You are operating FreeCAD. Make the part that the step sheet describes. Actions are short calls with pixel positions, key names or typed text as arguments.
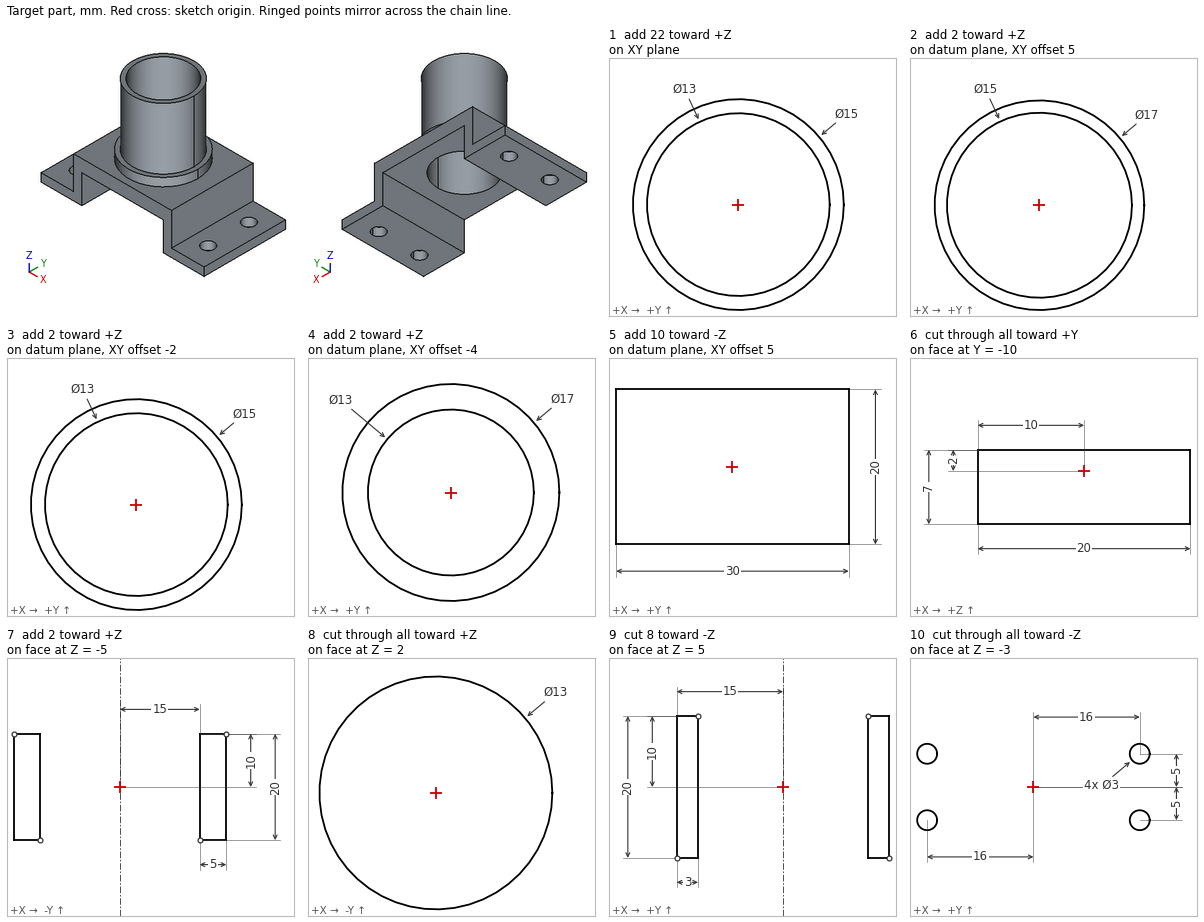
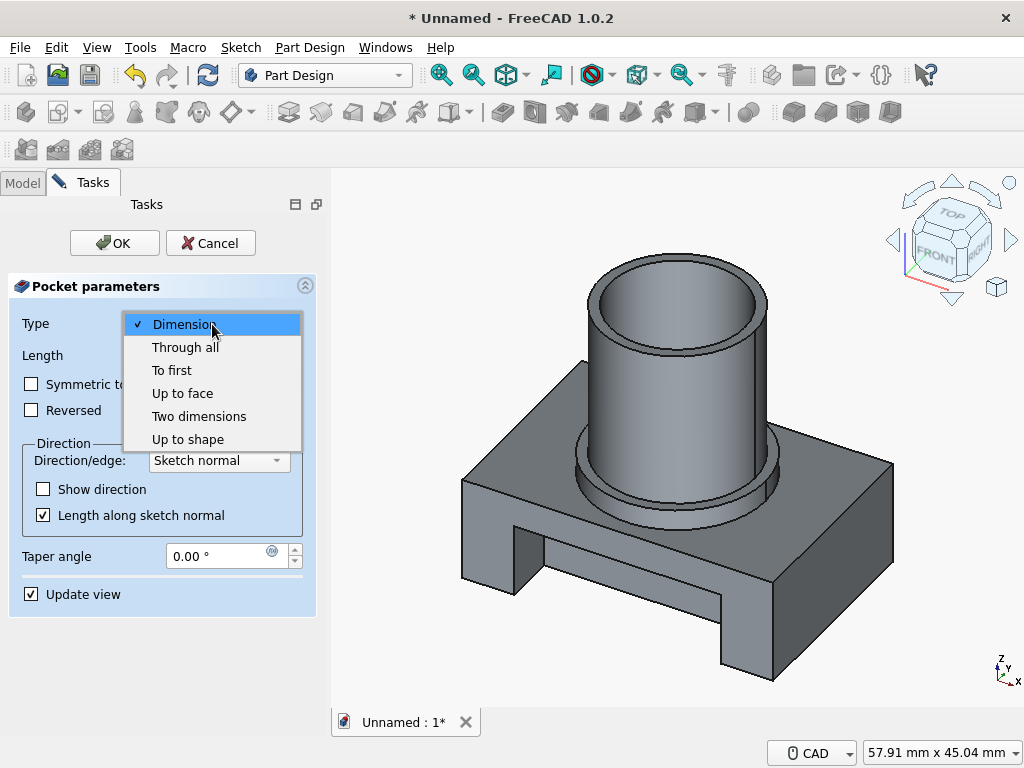
click(212, 348)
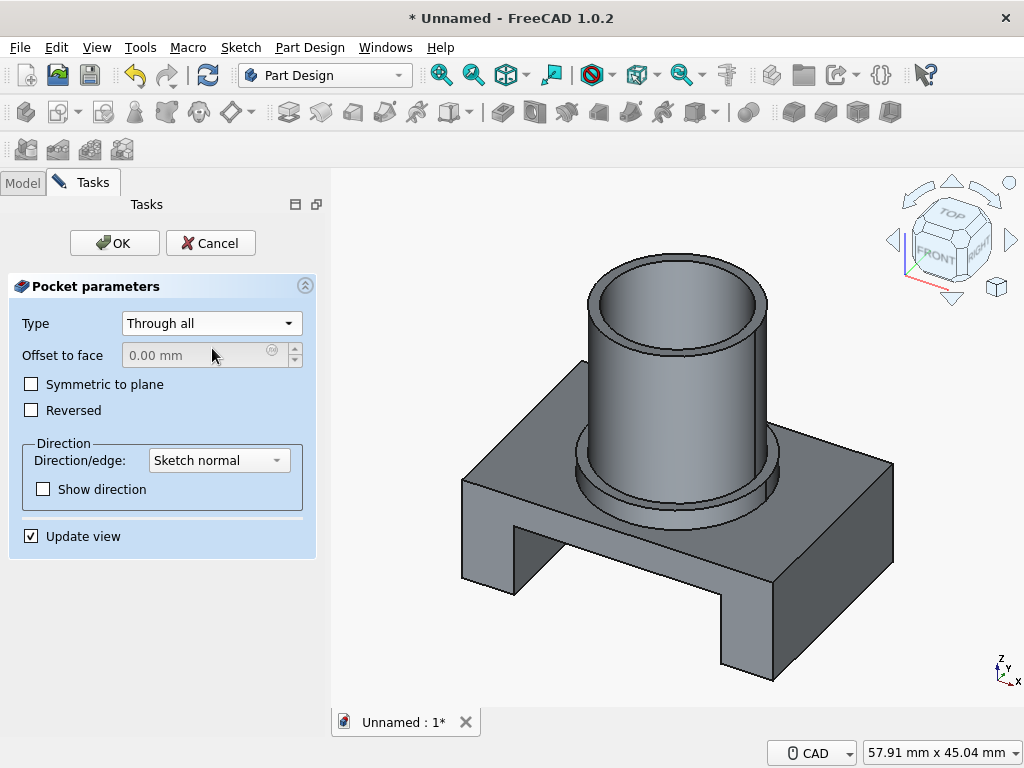
click(115, 243)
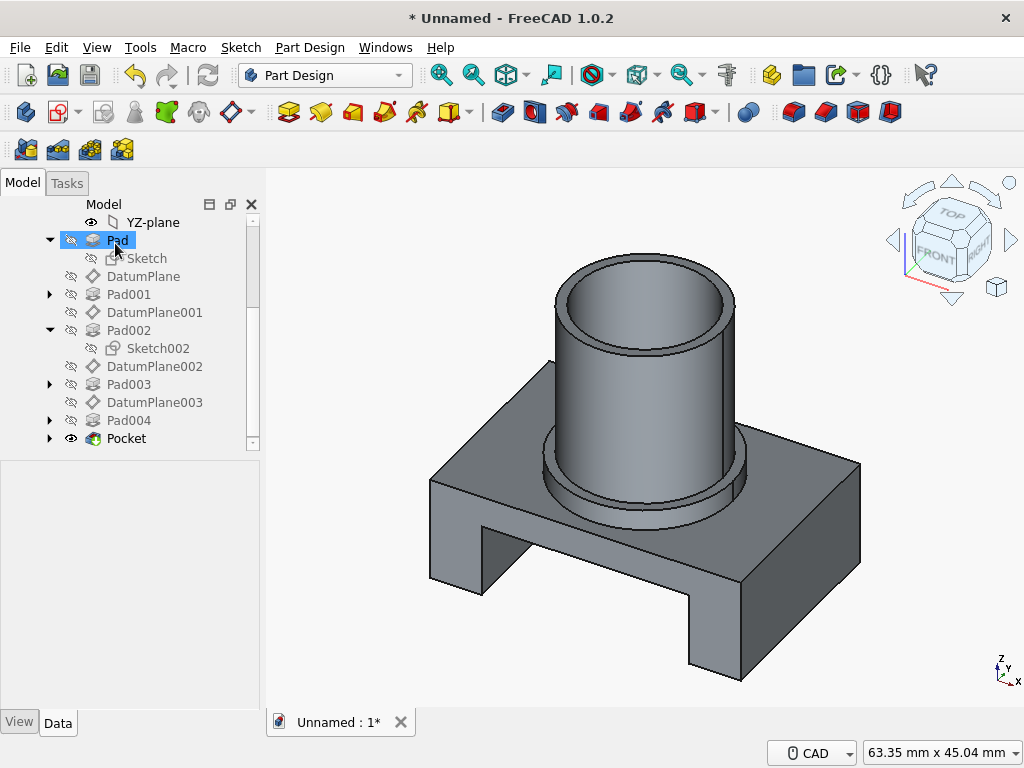
key(5)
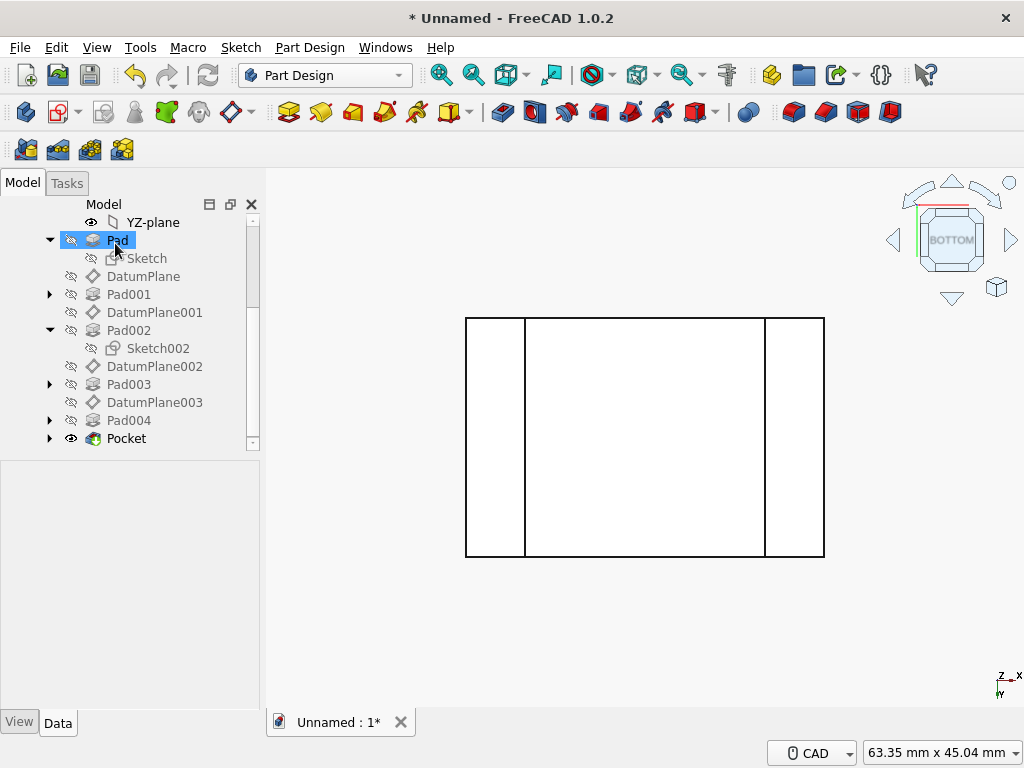
click(795, 505)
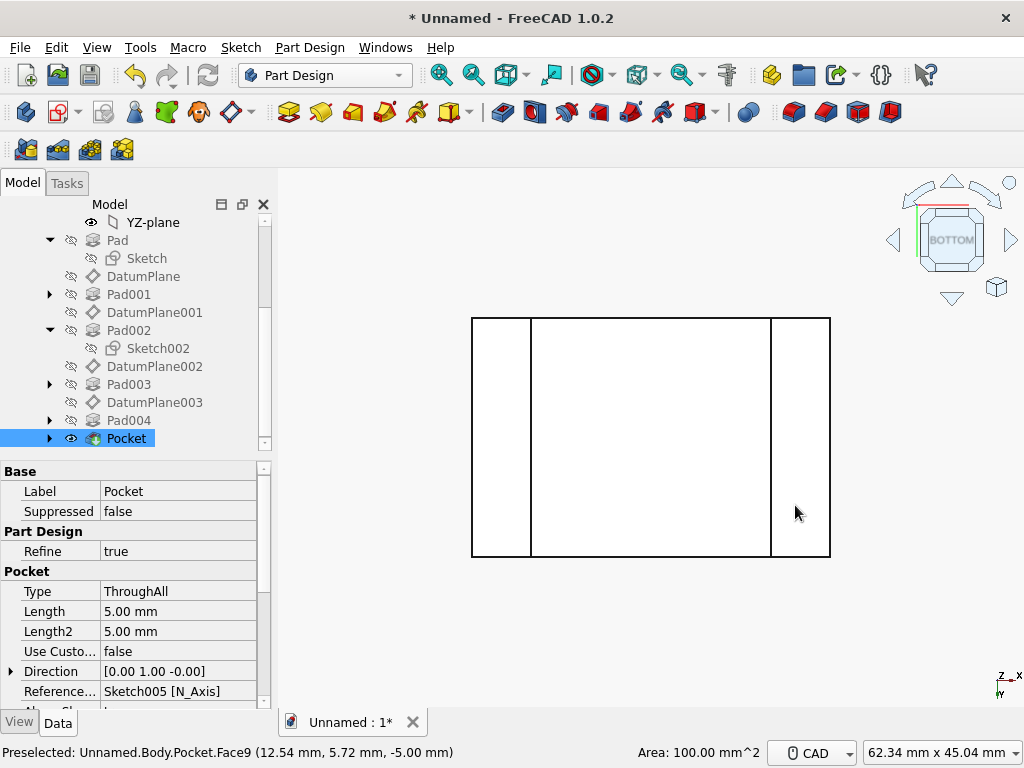
click(58, 112)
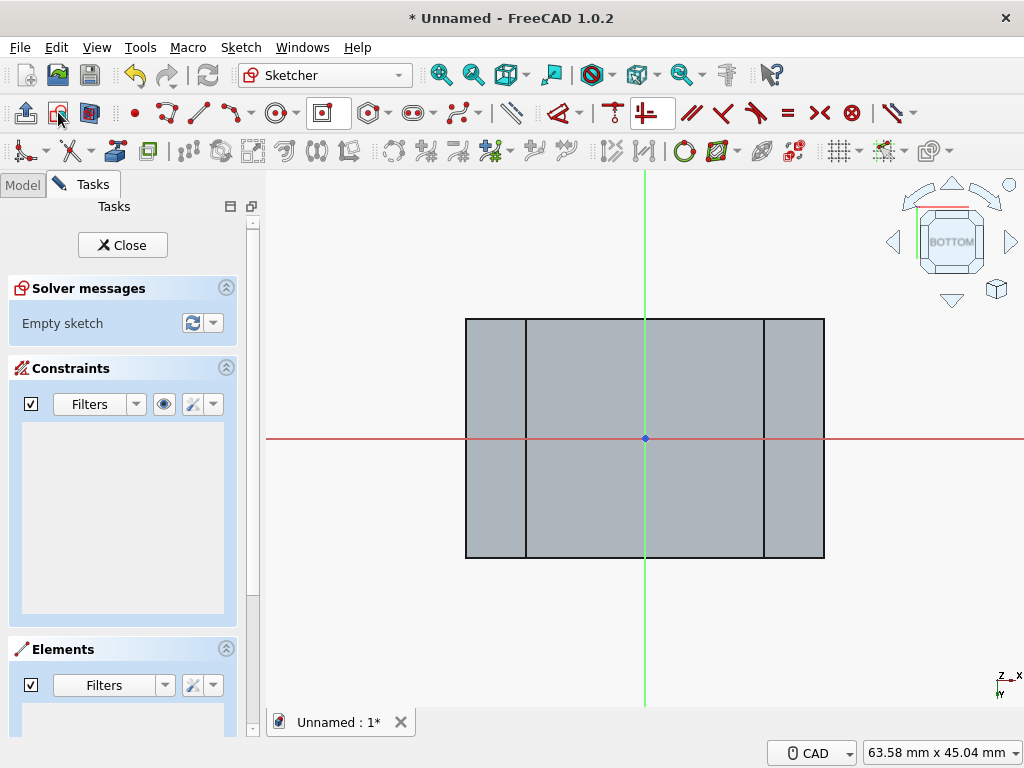
scroll(294, 439, down, 1)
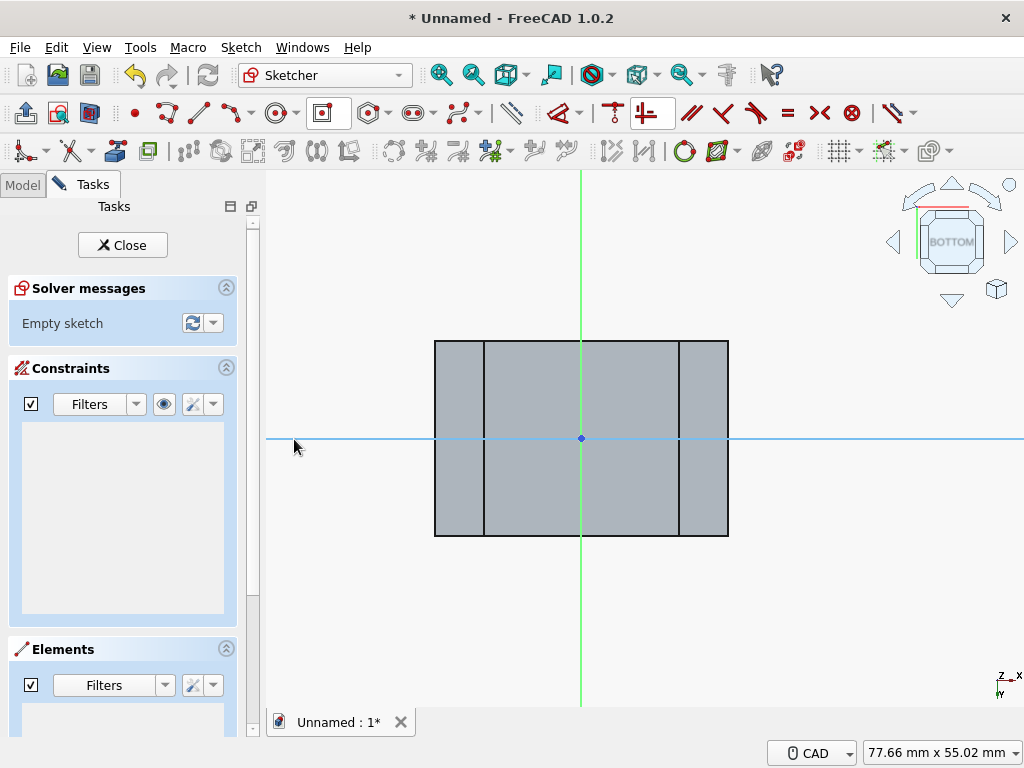
key(g)
key(r)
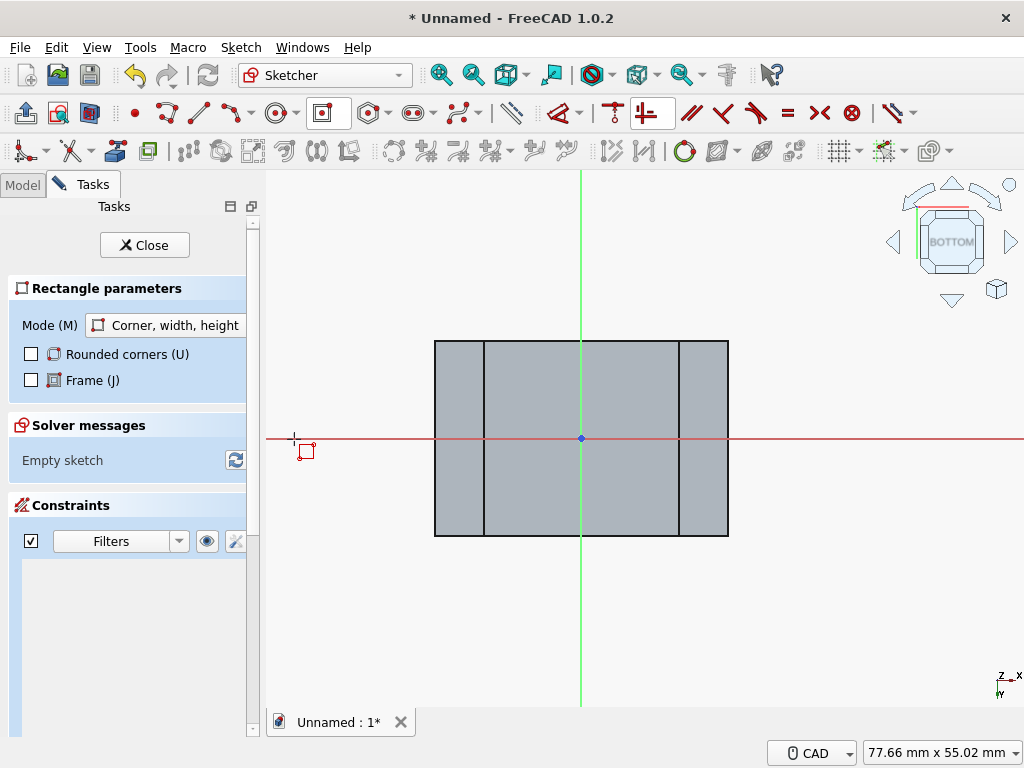
click(728, 341)
click(777, 536)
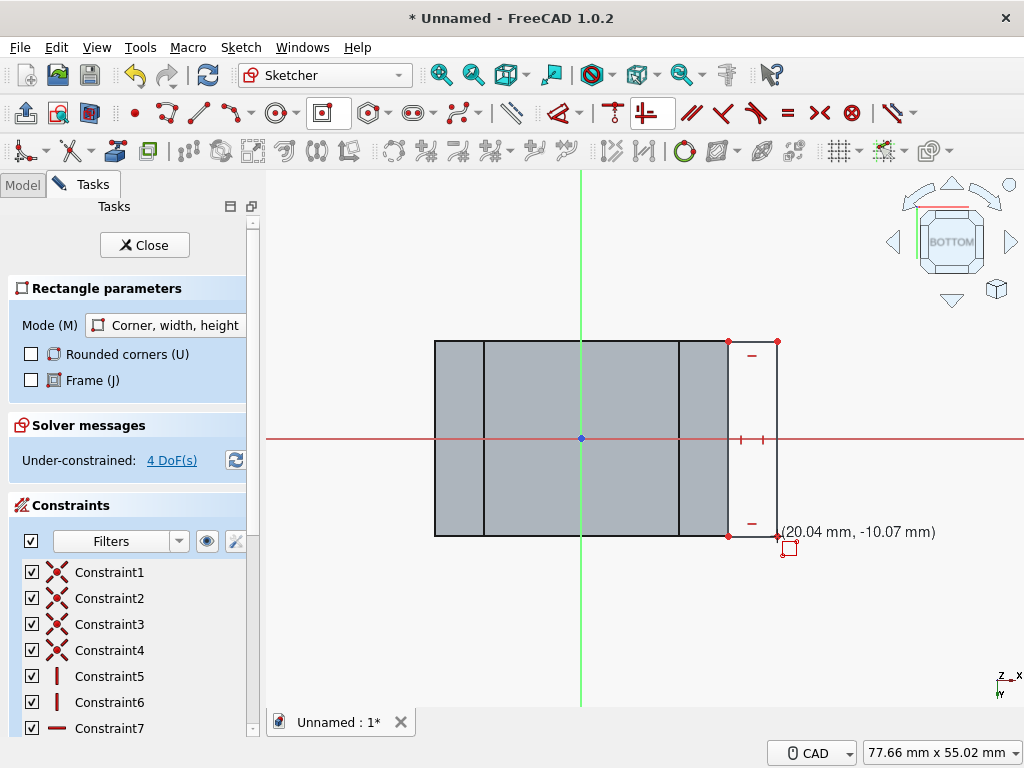
click(386, 341)
click(435, 536)
key(Escape)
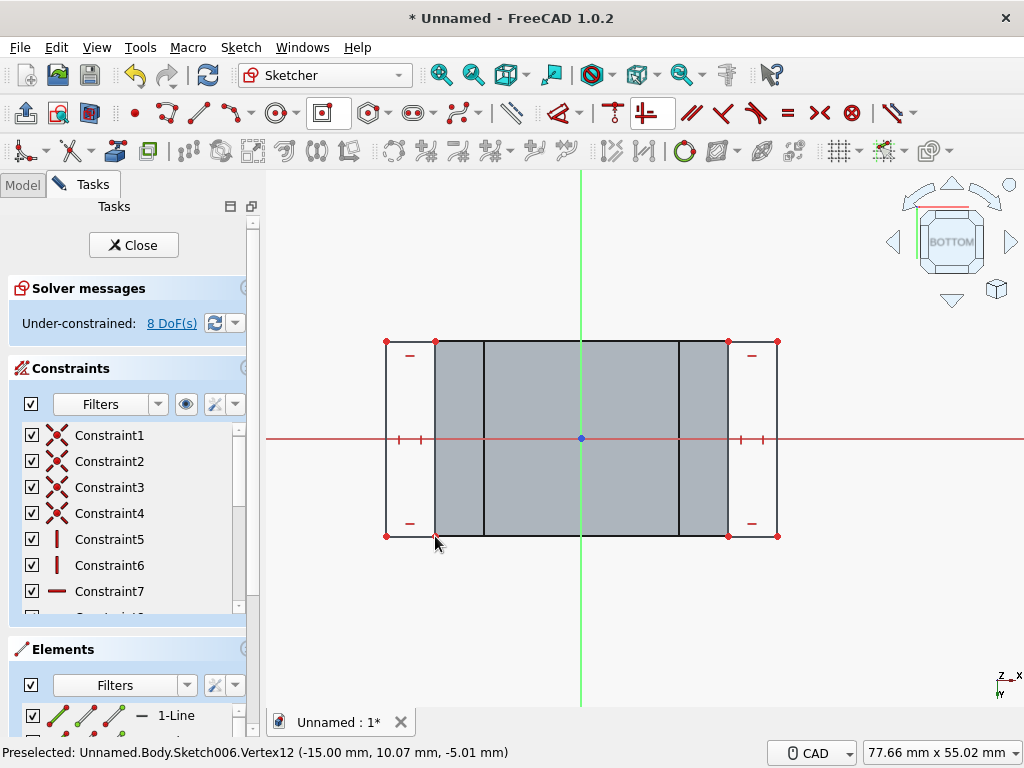
click(777, 342)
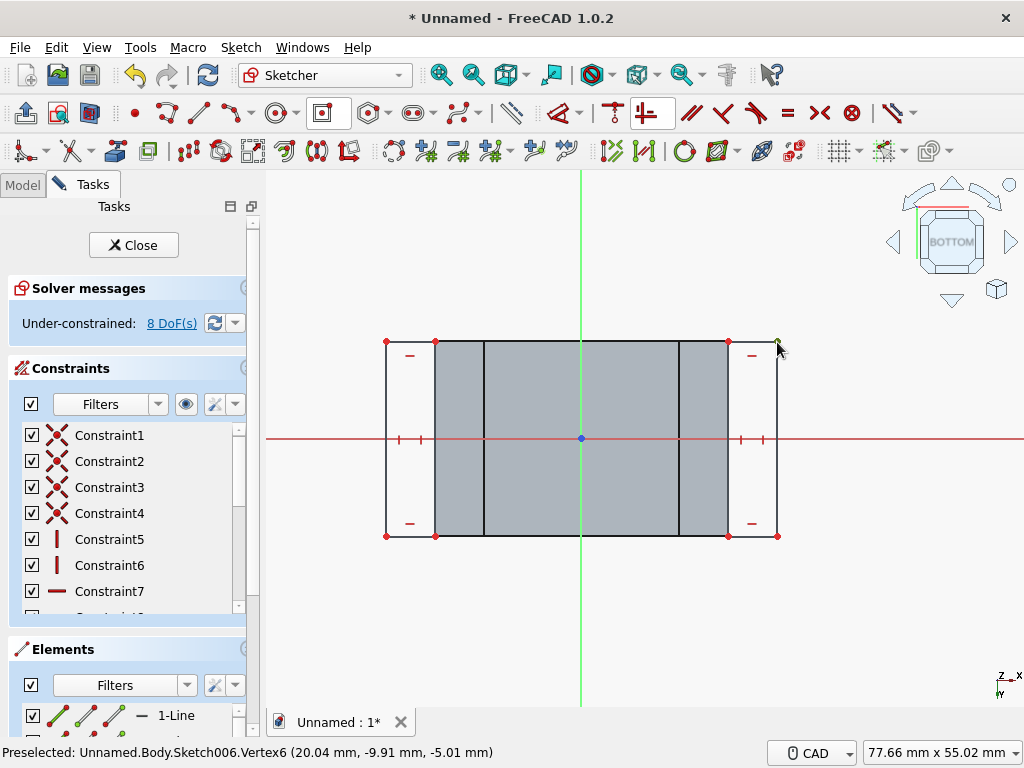
click(386, 342)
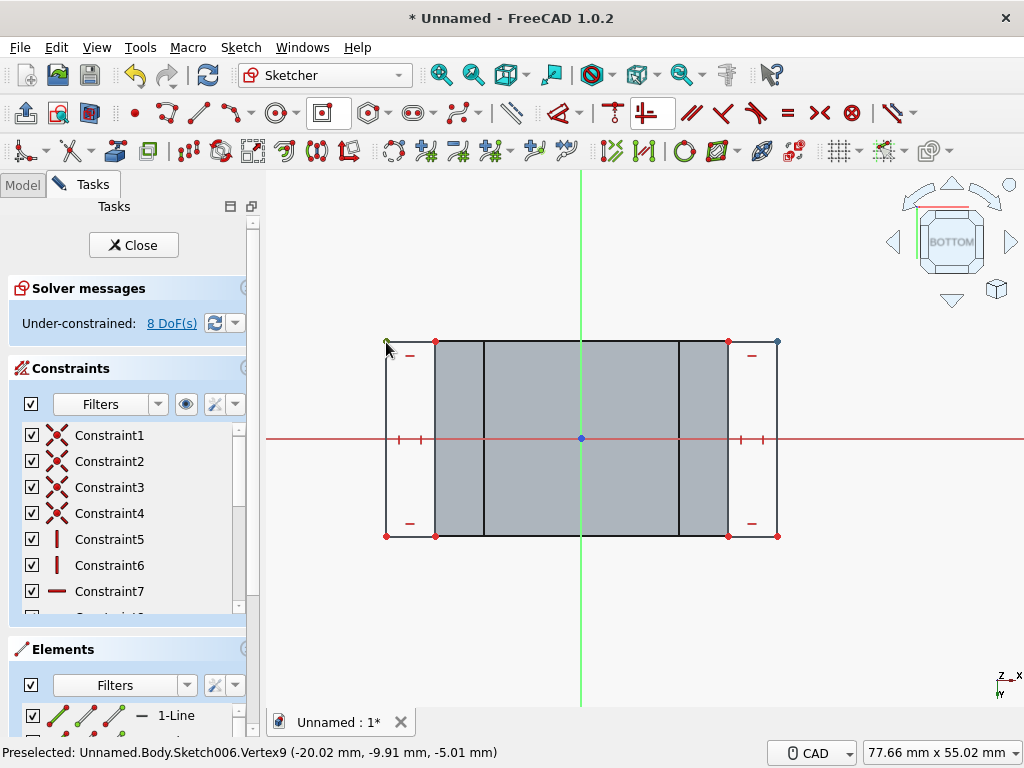
click(581, 645)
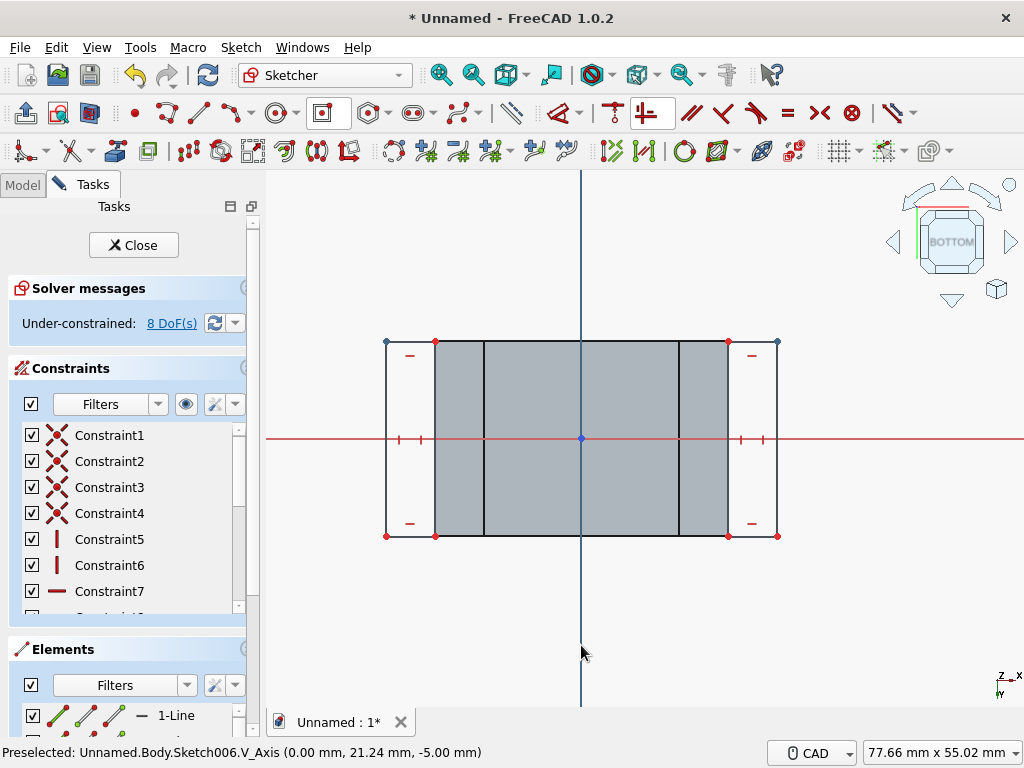
key(s)